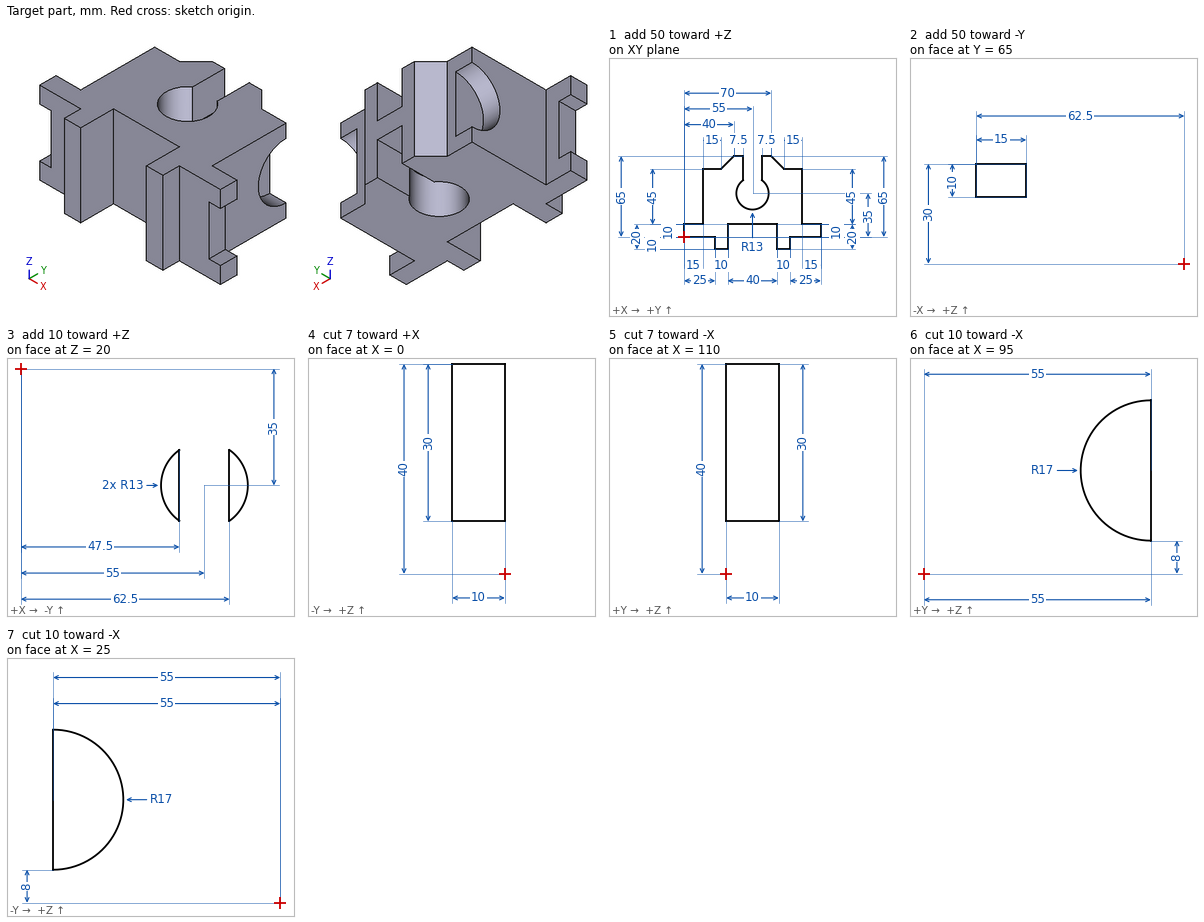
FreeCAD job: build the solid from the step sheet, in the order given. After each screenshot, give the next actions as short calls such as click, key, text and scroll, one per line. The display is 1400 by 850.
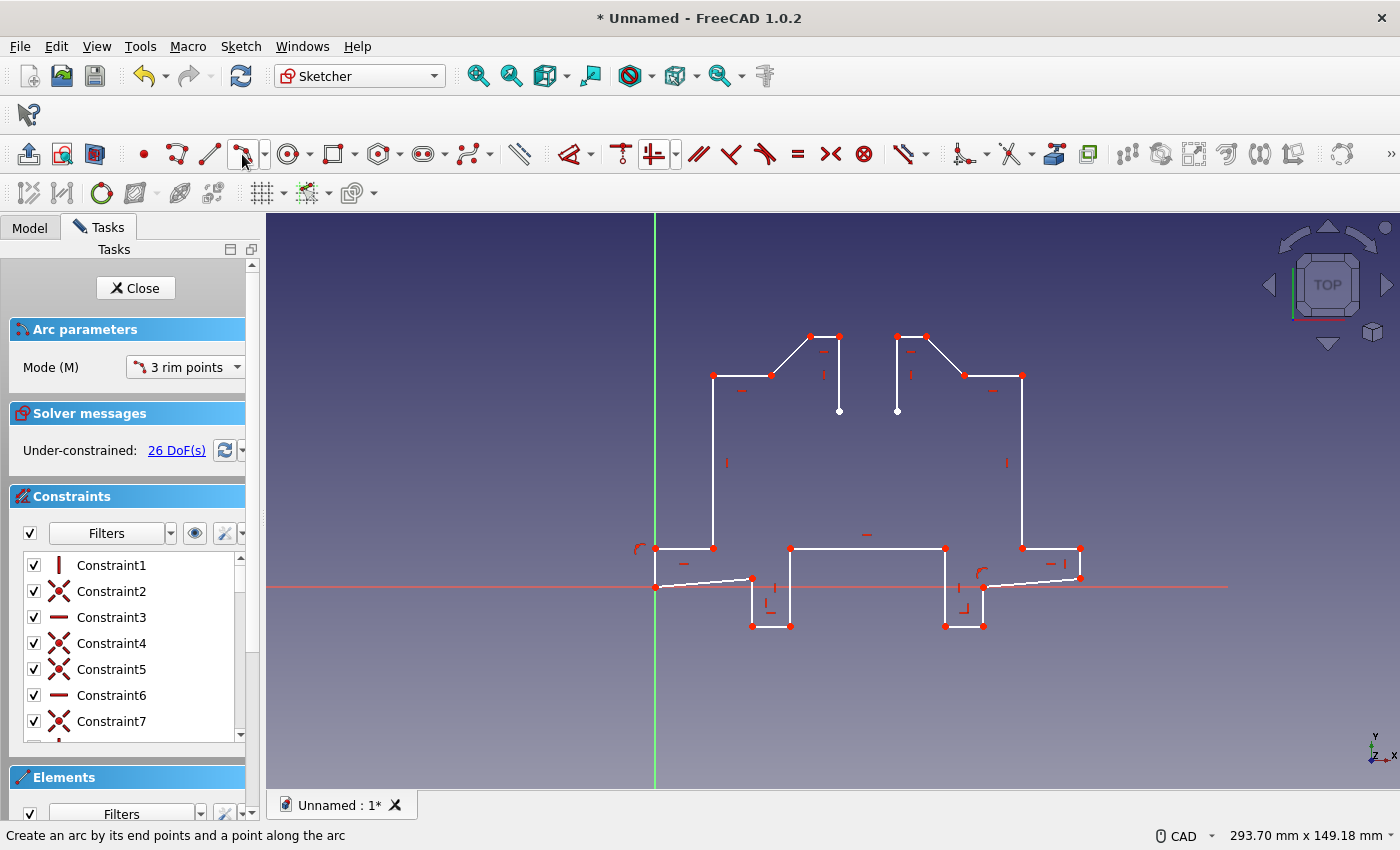
click(897, 412)
click(839, 412)
click(868, 502)
key(Escape)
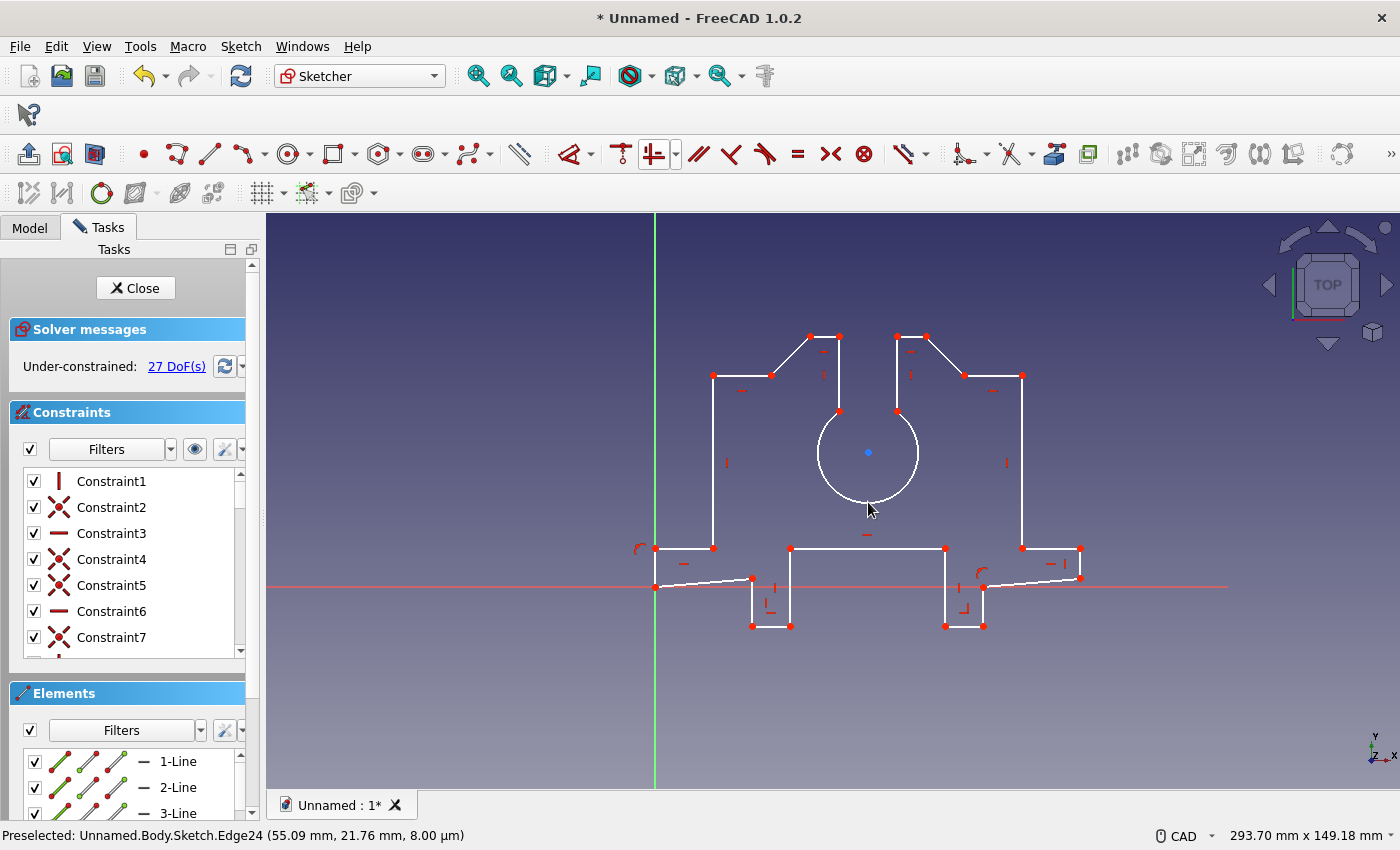
click(684, 585)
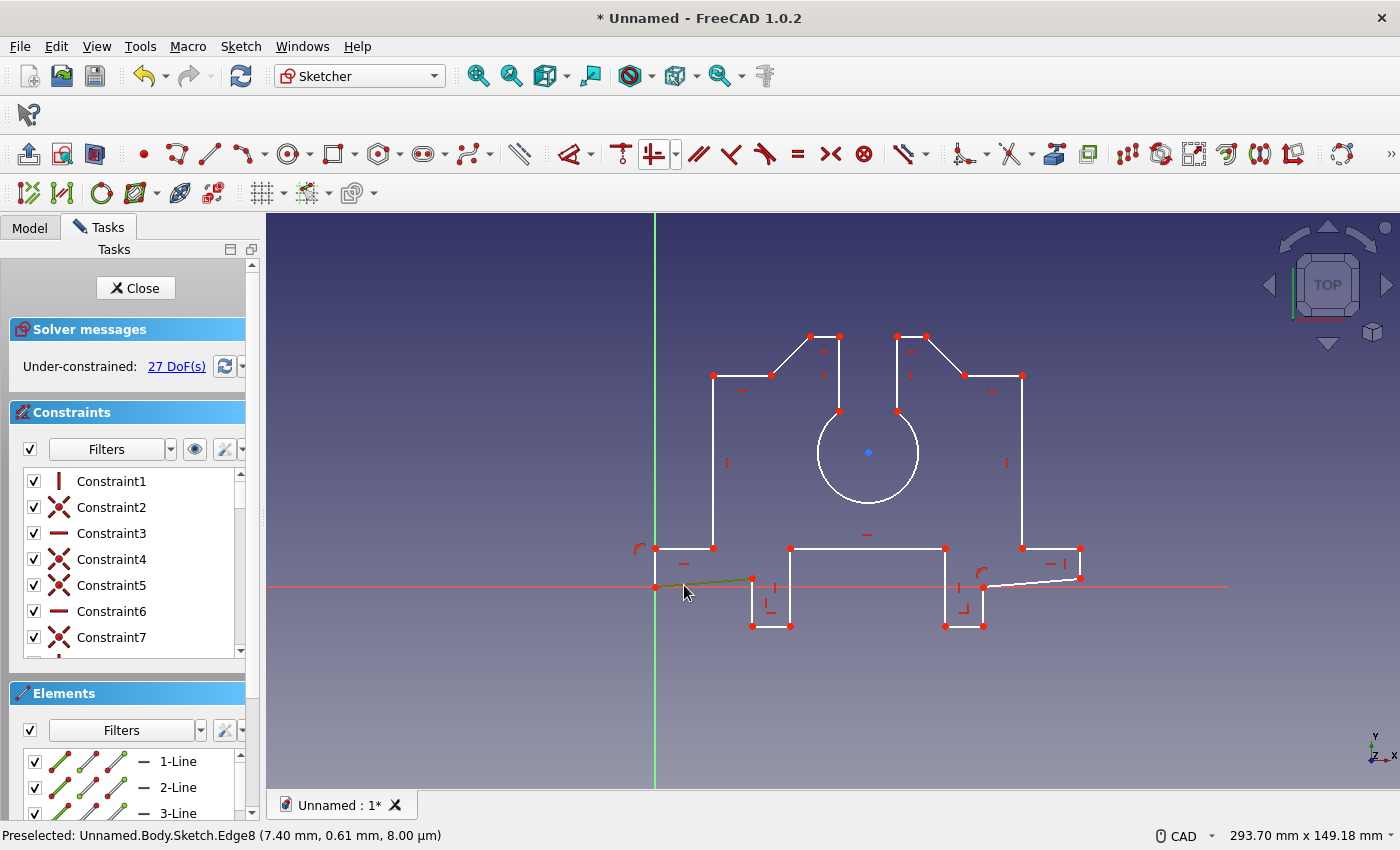
click(676, 154)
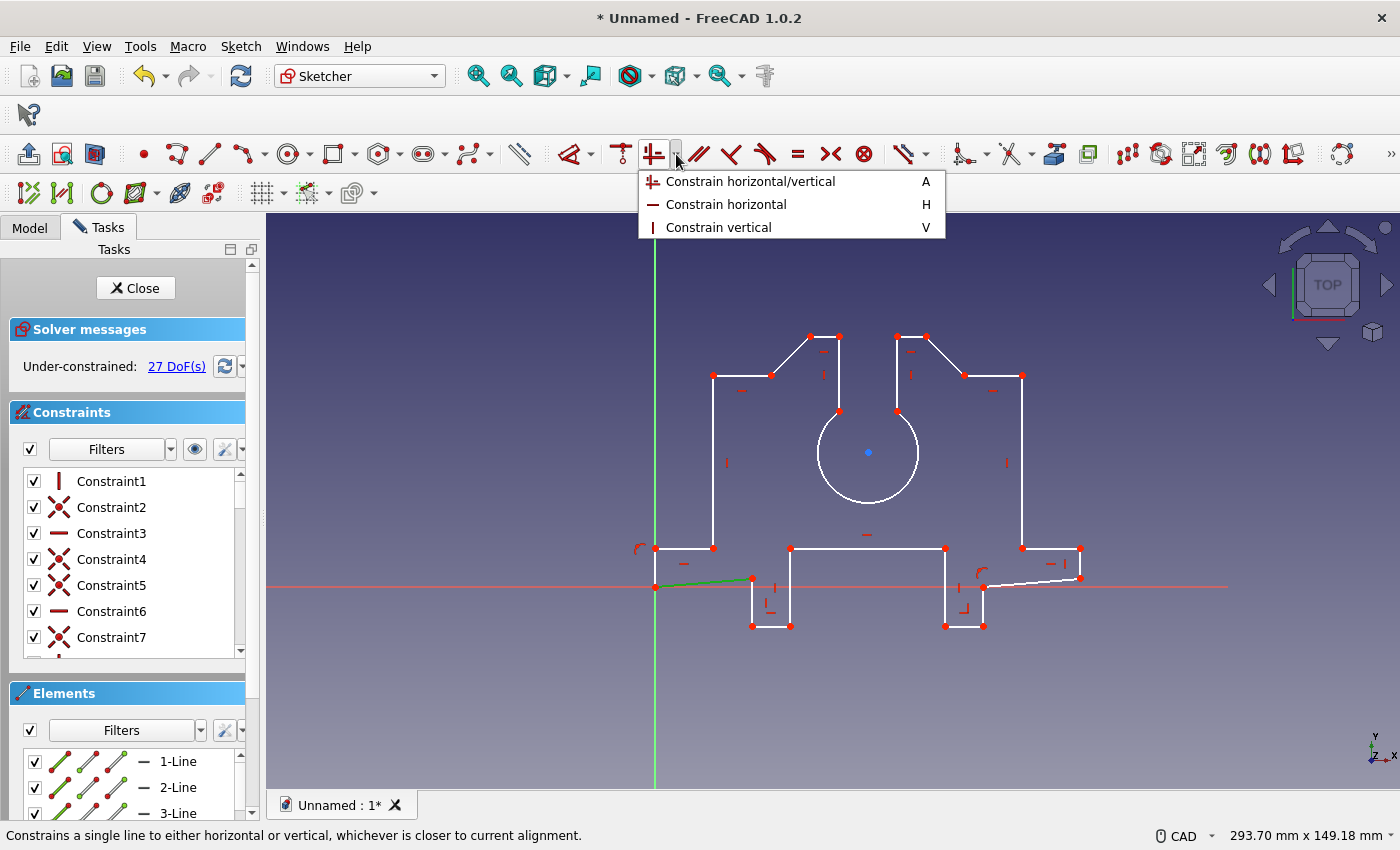
click(792, 204)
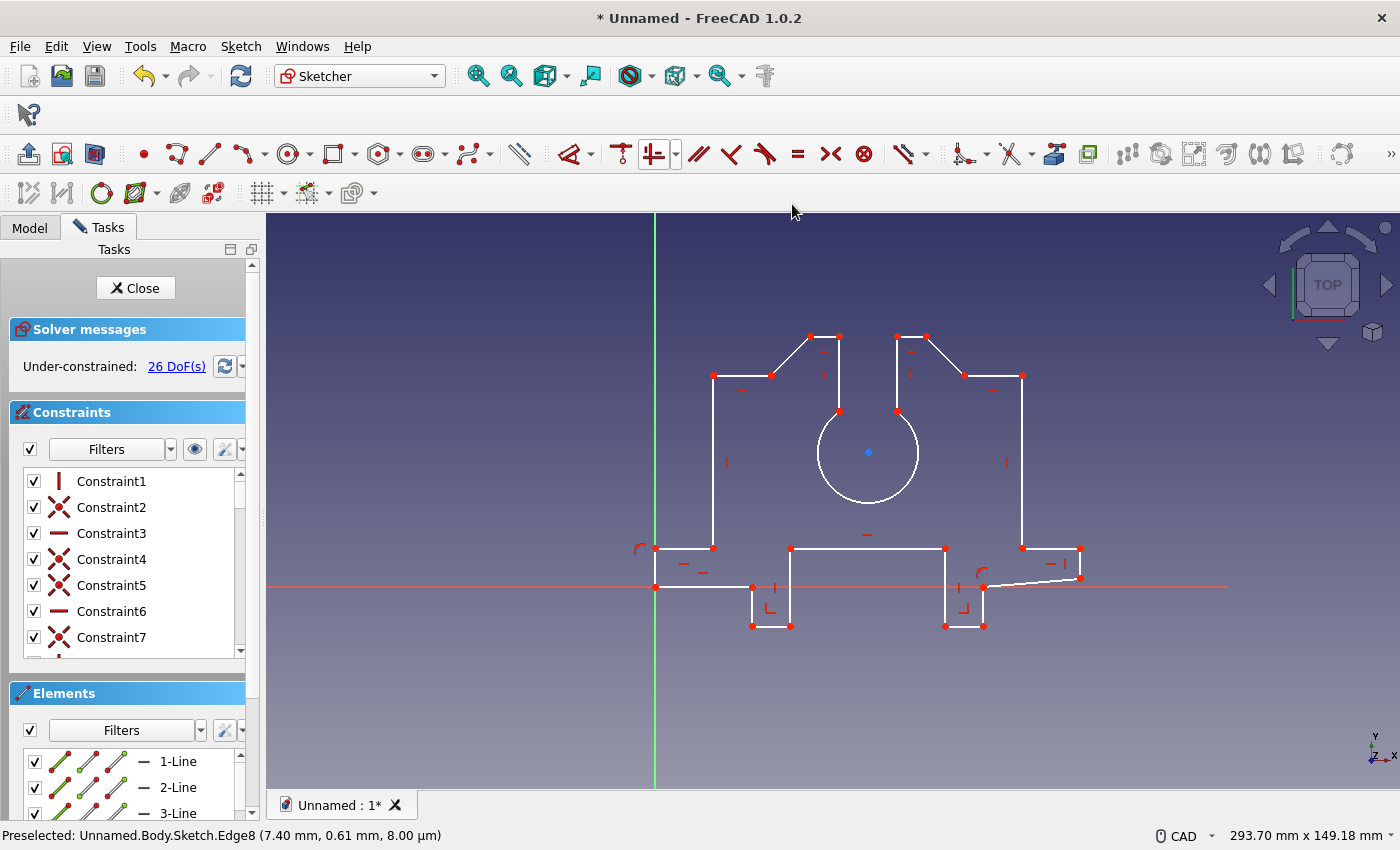
click(1012, 585)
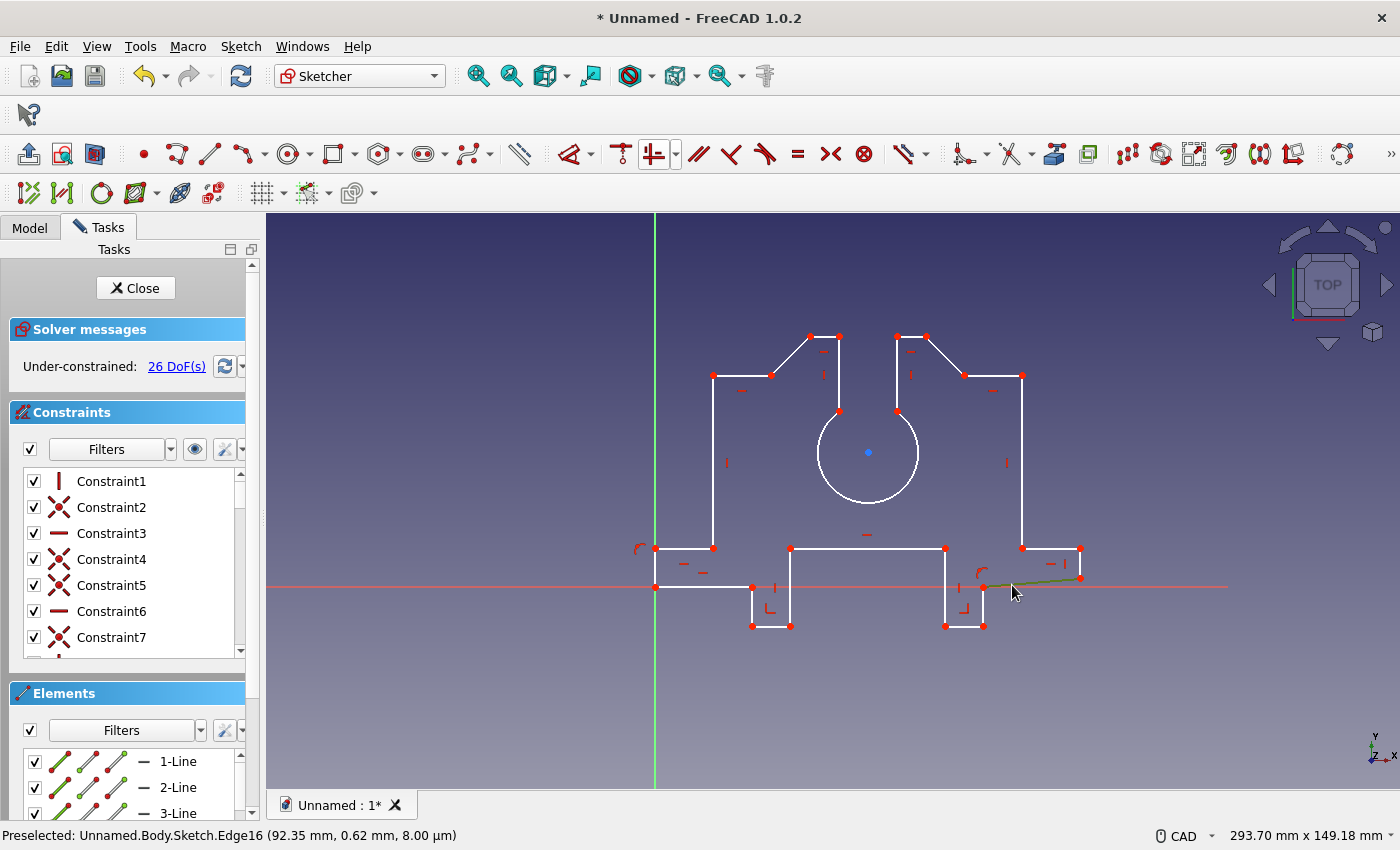
key(h)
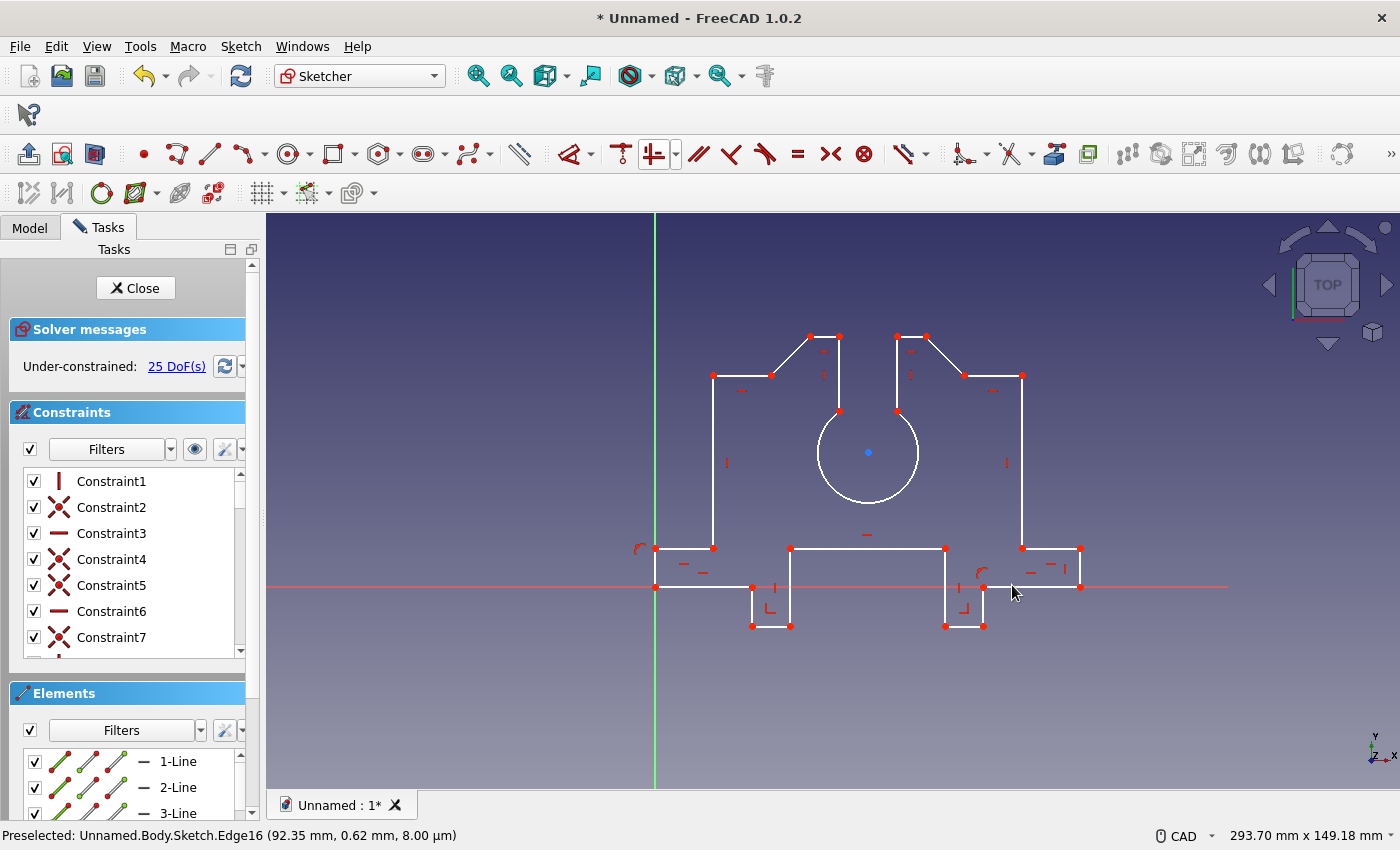
click(568, 154)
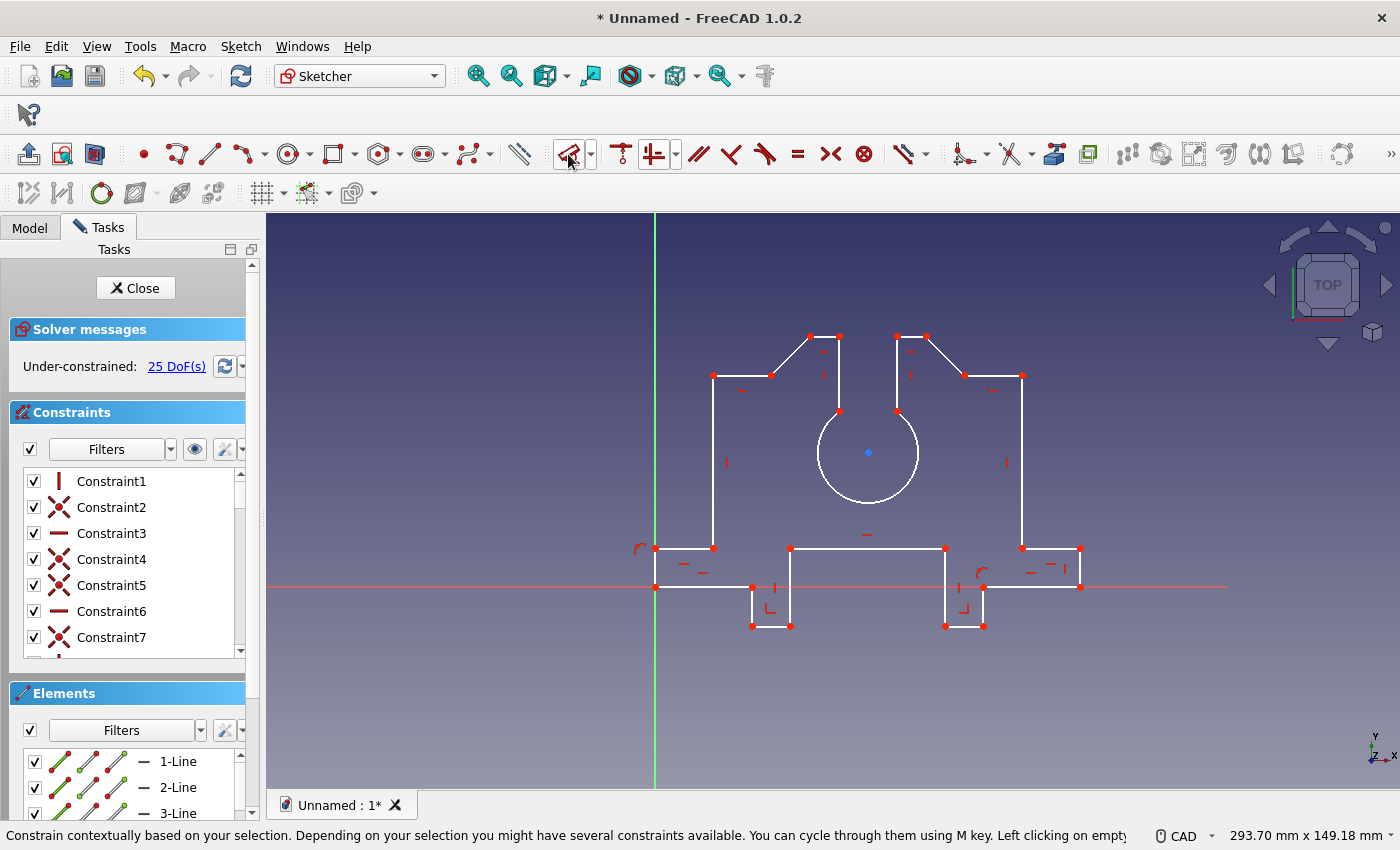
click(826, 480)
click(799, 497)